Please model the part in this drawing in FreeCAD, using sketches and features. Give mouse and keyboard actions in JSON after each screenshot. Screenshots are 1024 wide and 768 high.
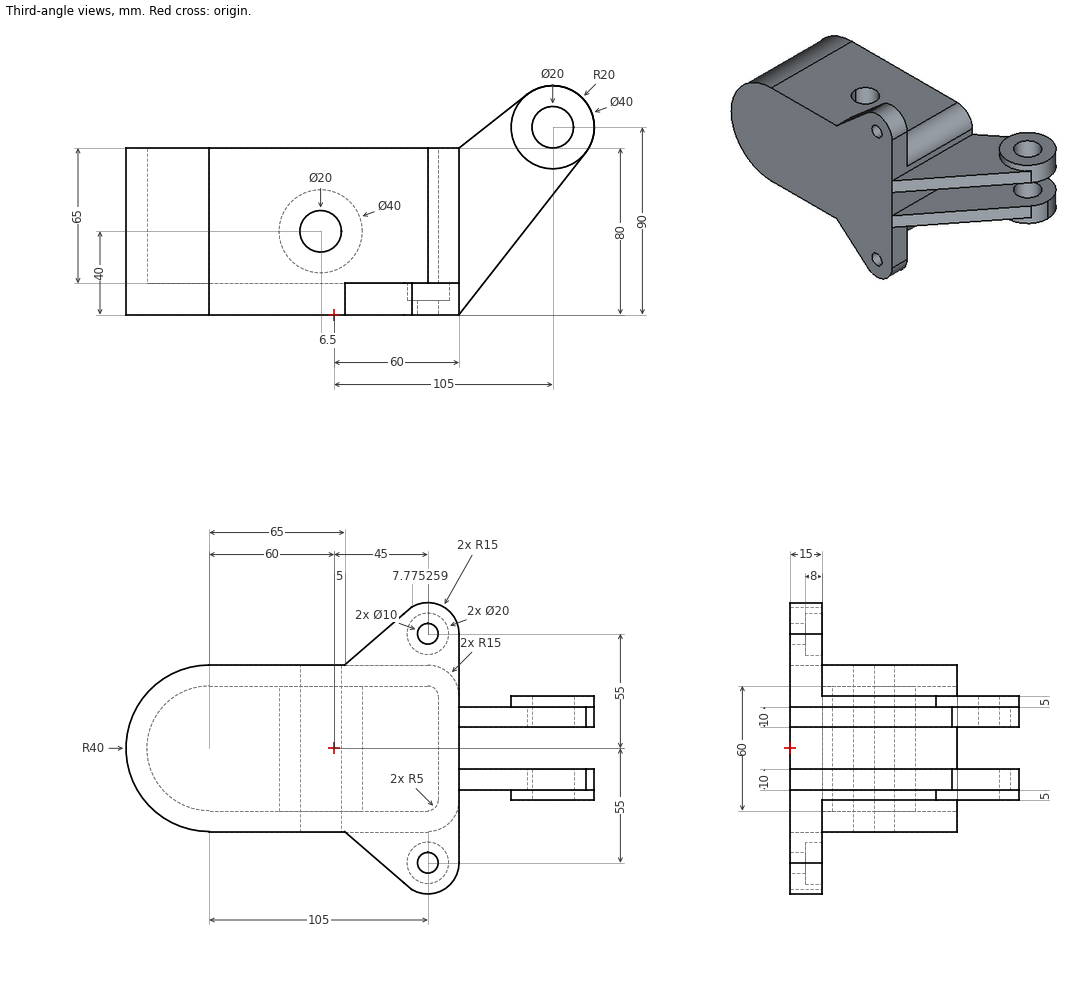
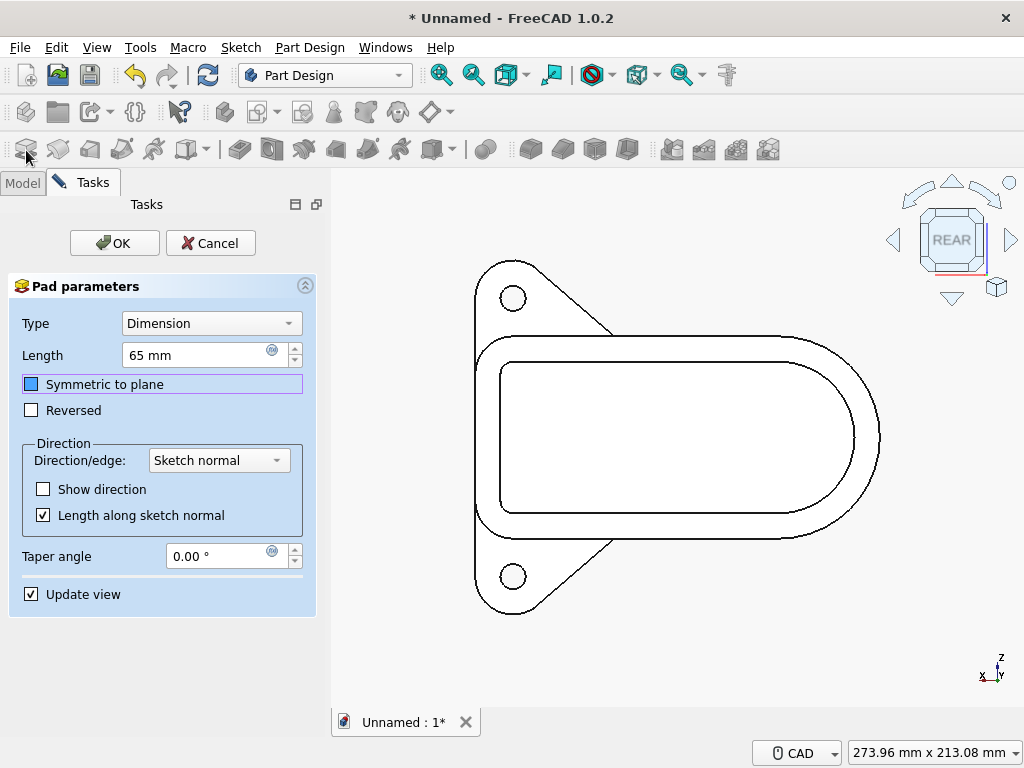
{"action": "left_click", "coordinate": [115, 243]}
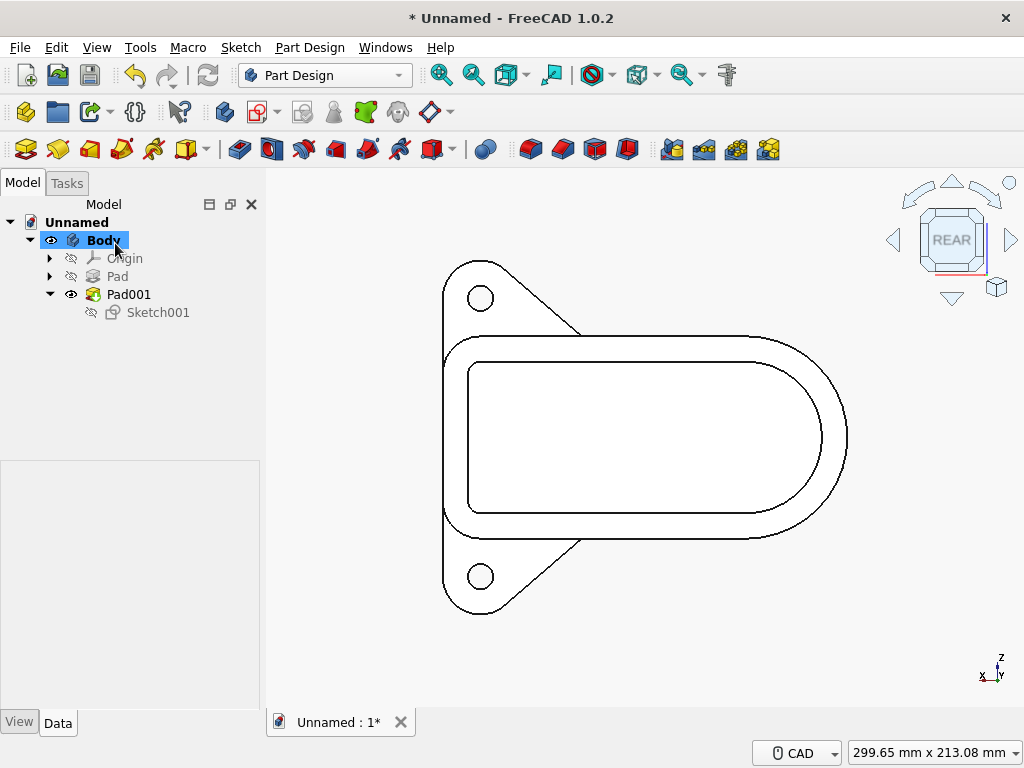
{"action": "left_click", "coordinate": [594, 436]}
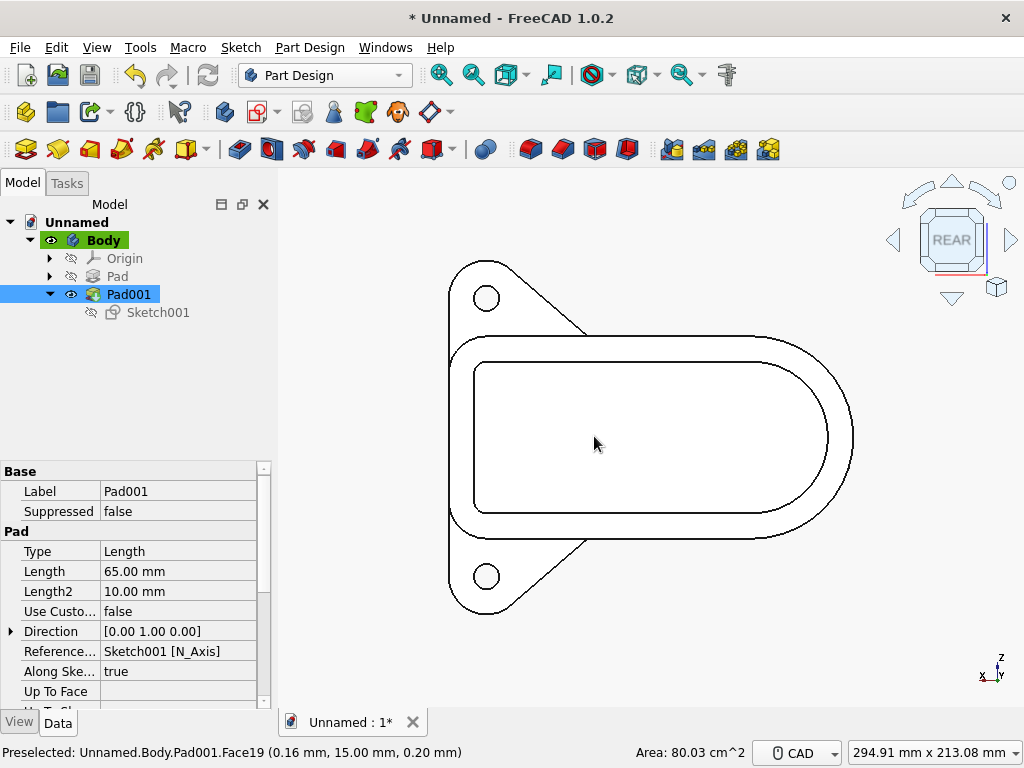
{"action": "left_click", "coordinate": [258, 112]}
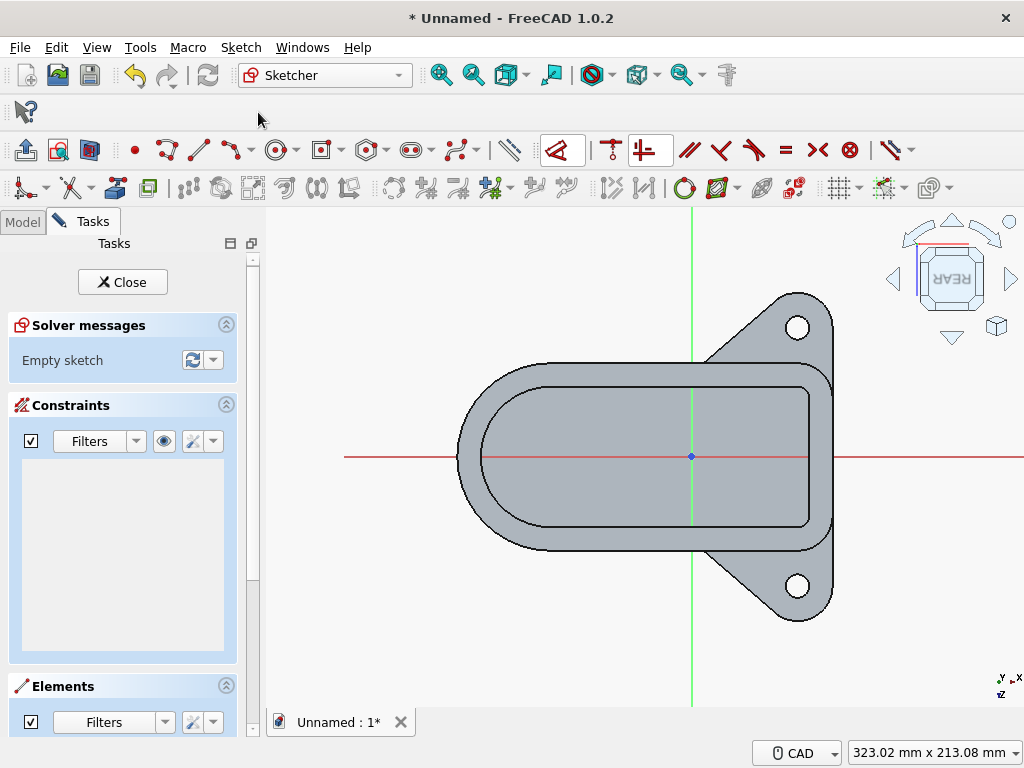
{"action": "left_click", "coordinate": [90, 150]}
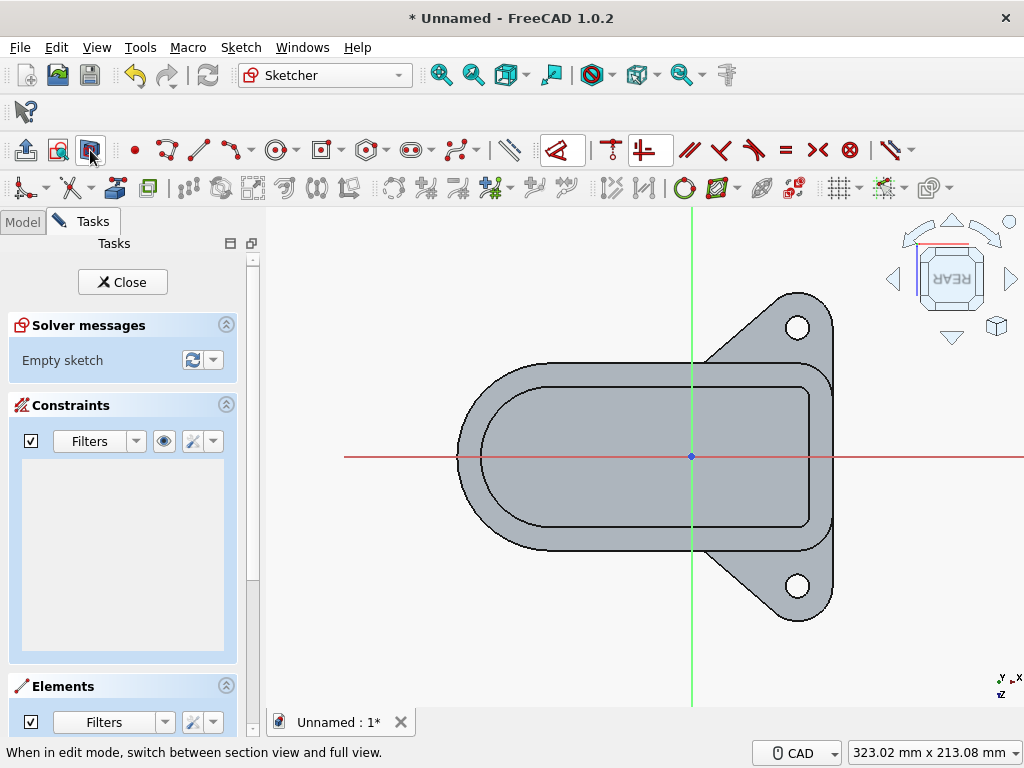
{"action": "left_click", "coordinate": [276, 150]}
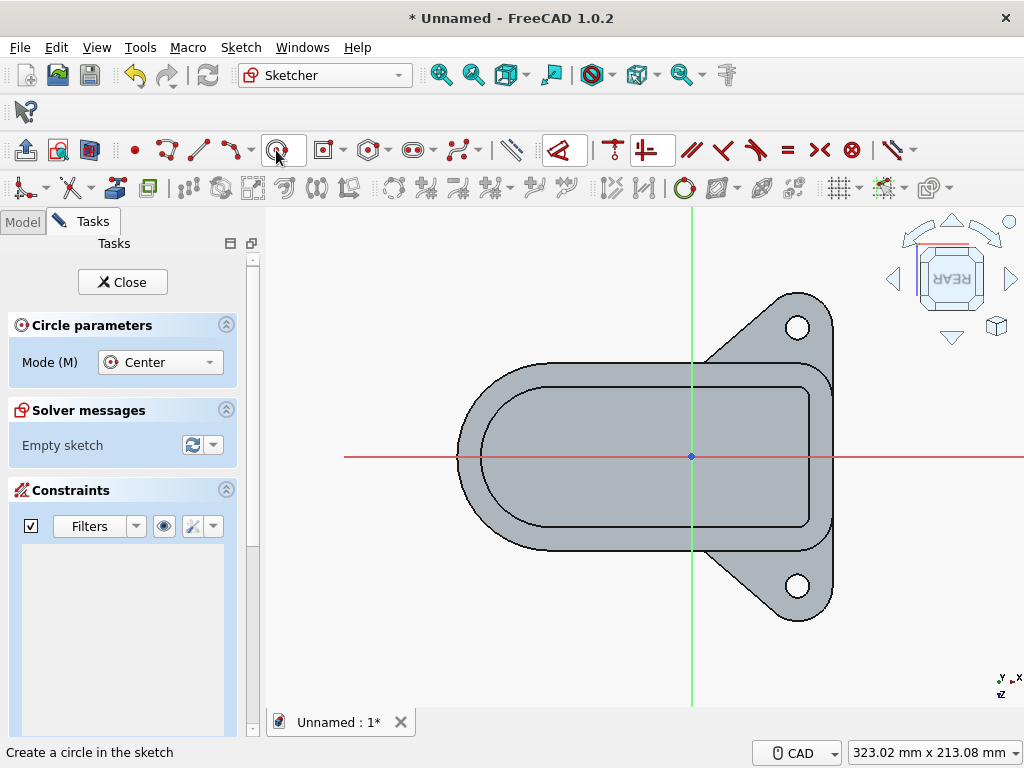
{"action": "left_click", "coordinate": [798, 586]}
{"action": "left_click", "coordinate": [814, 569]}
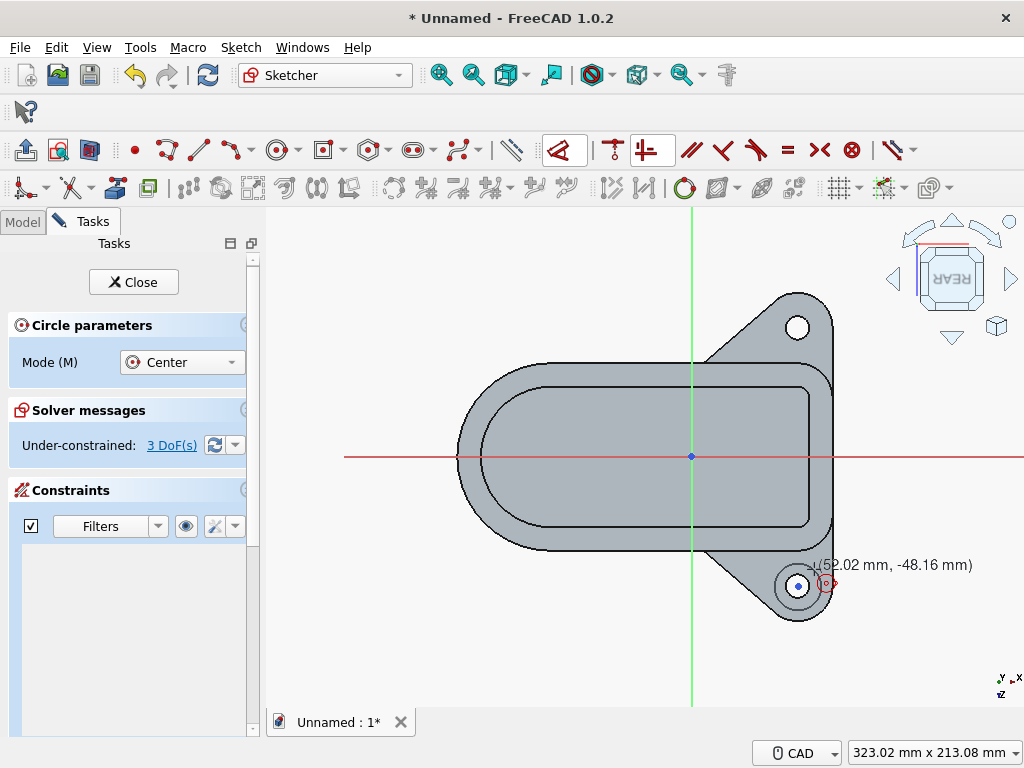
{"action": "left_click", "coordinate": [798, 328]}
{"action": "left_click", "coordinate": [814, 311]}
{"action": "key", "text": "Escape"}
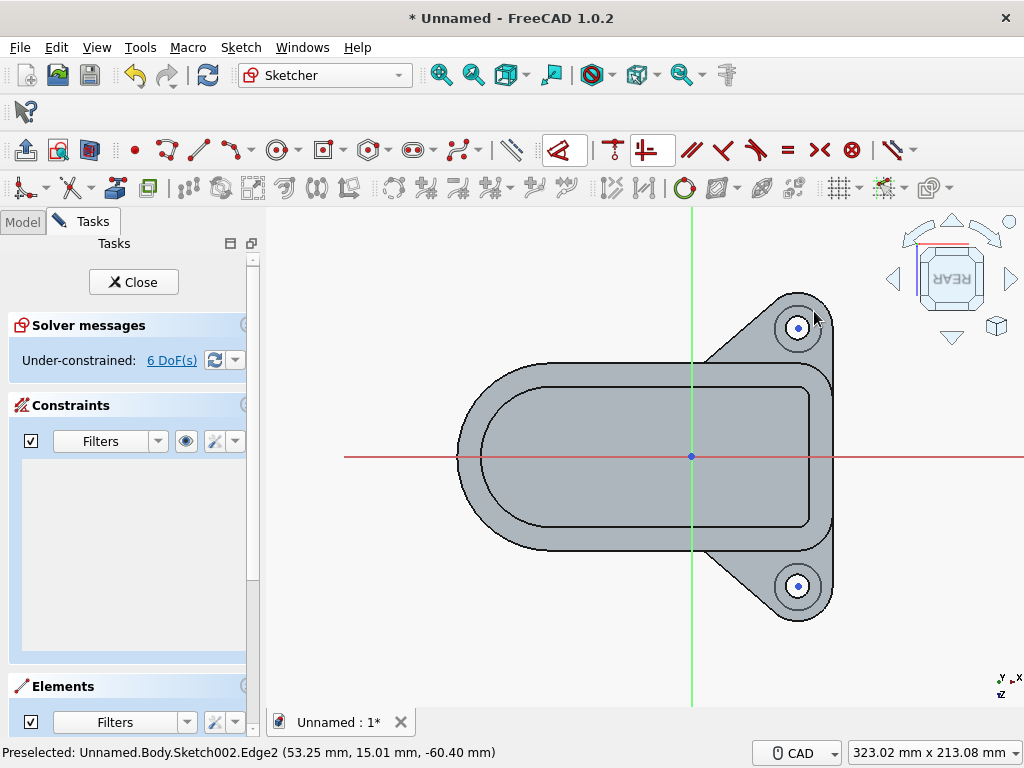
{"action": "left_click", "coordinate": [814, 570]}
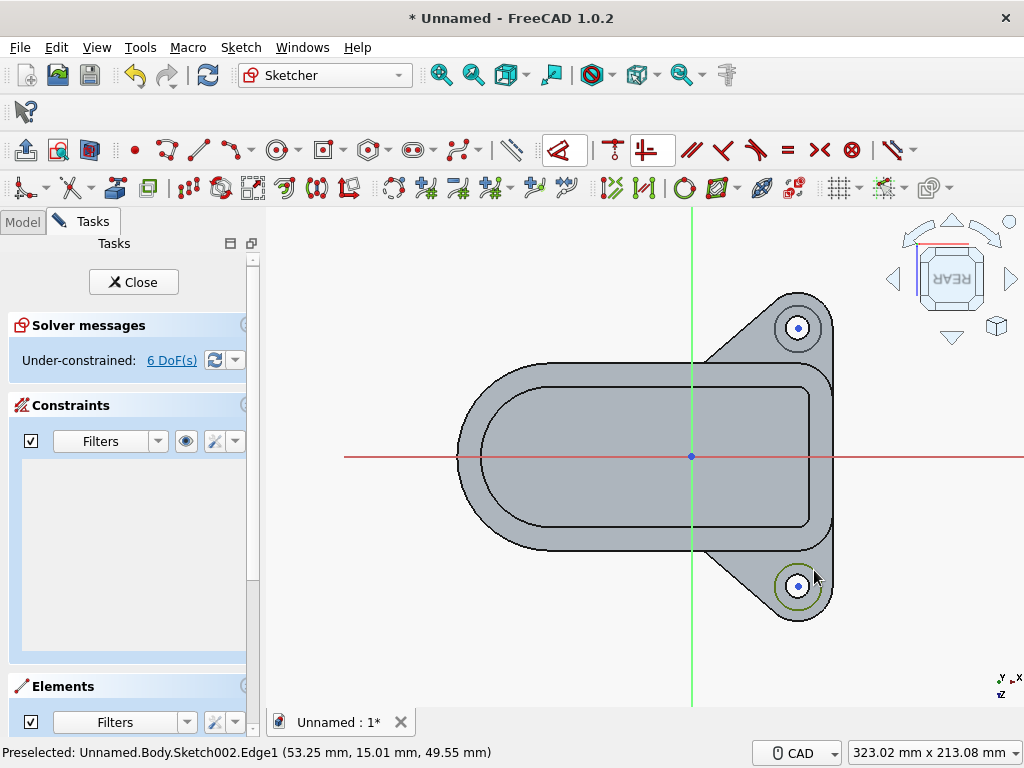
{"action": "left_click", "coordinate": [814, 312]}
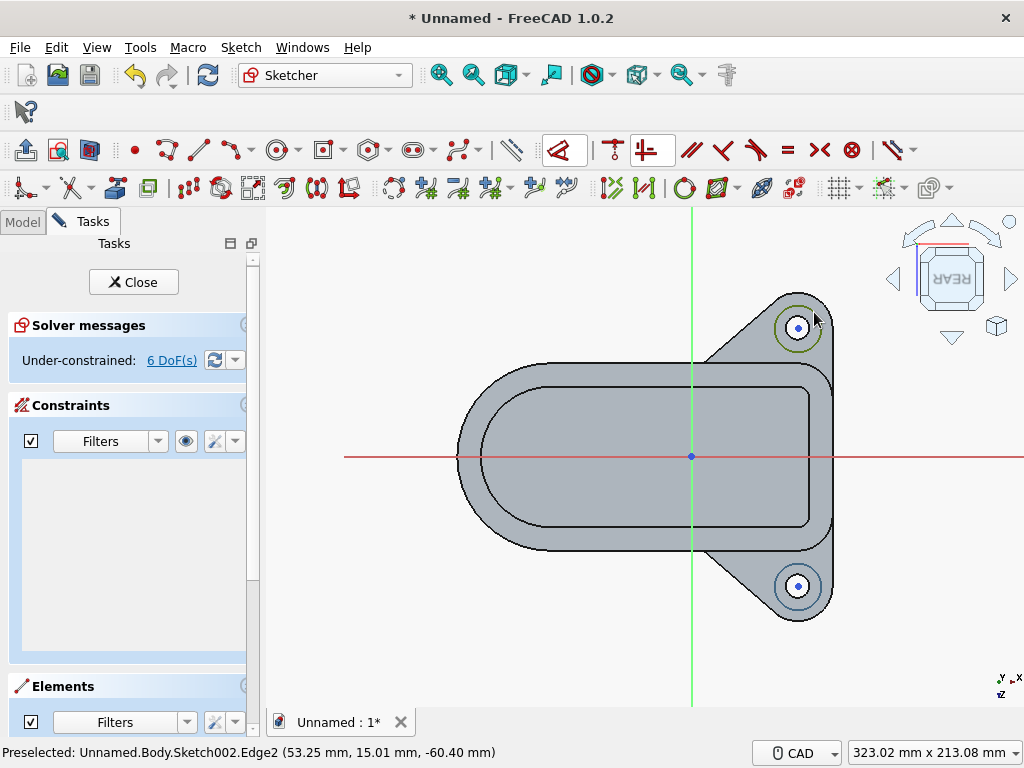
{"action": "left_click", "coordinate": [788, 150]}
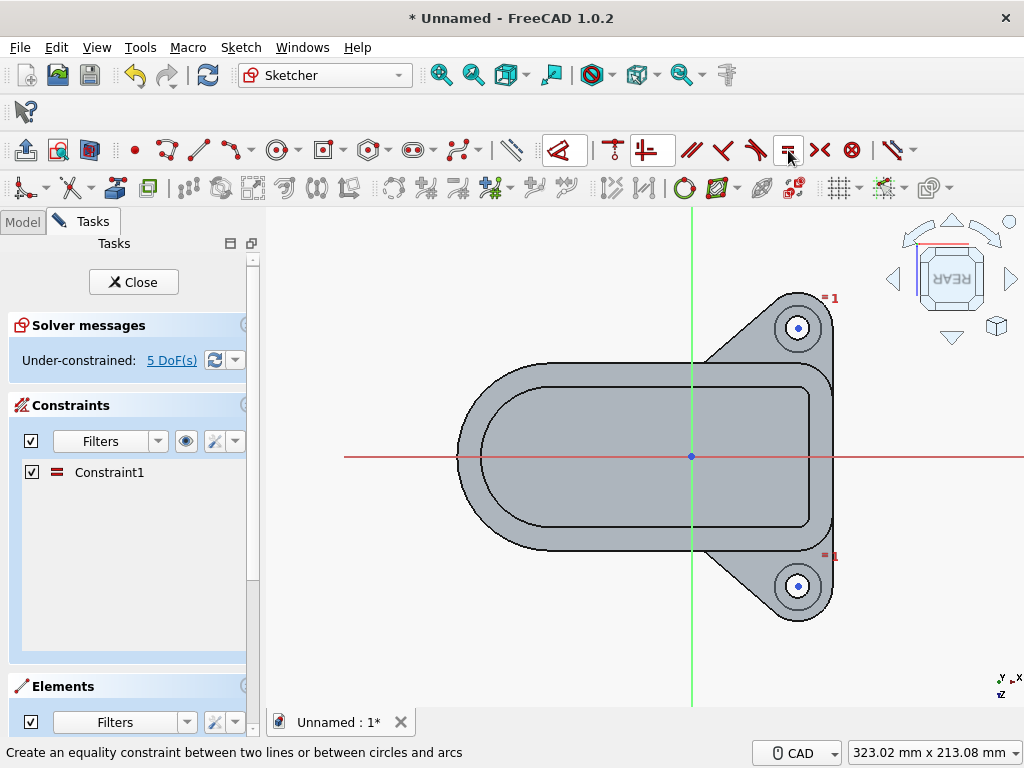
{"action": "left_click", "coordinate": [798, 587]}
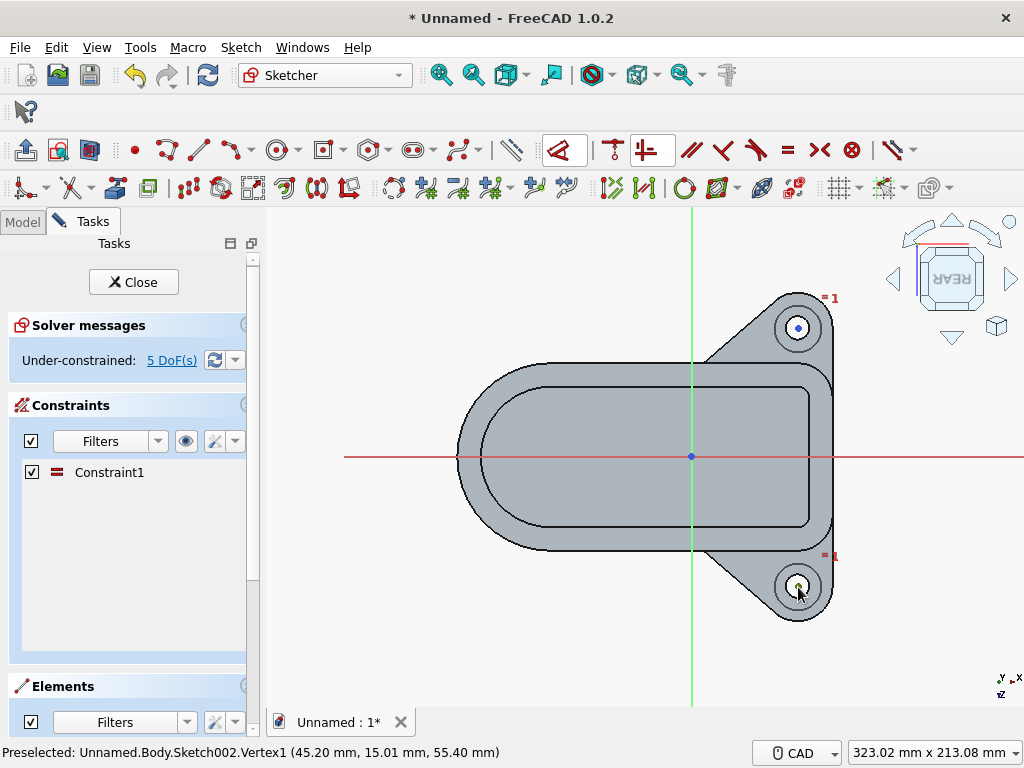
{"action": "left_click", "coordinate": [798, 329]}